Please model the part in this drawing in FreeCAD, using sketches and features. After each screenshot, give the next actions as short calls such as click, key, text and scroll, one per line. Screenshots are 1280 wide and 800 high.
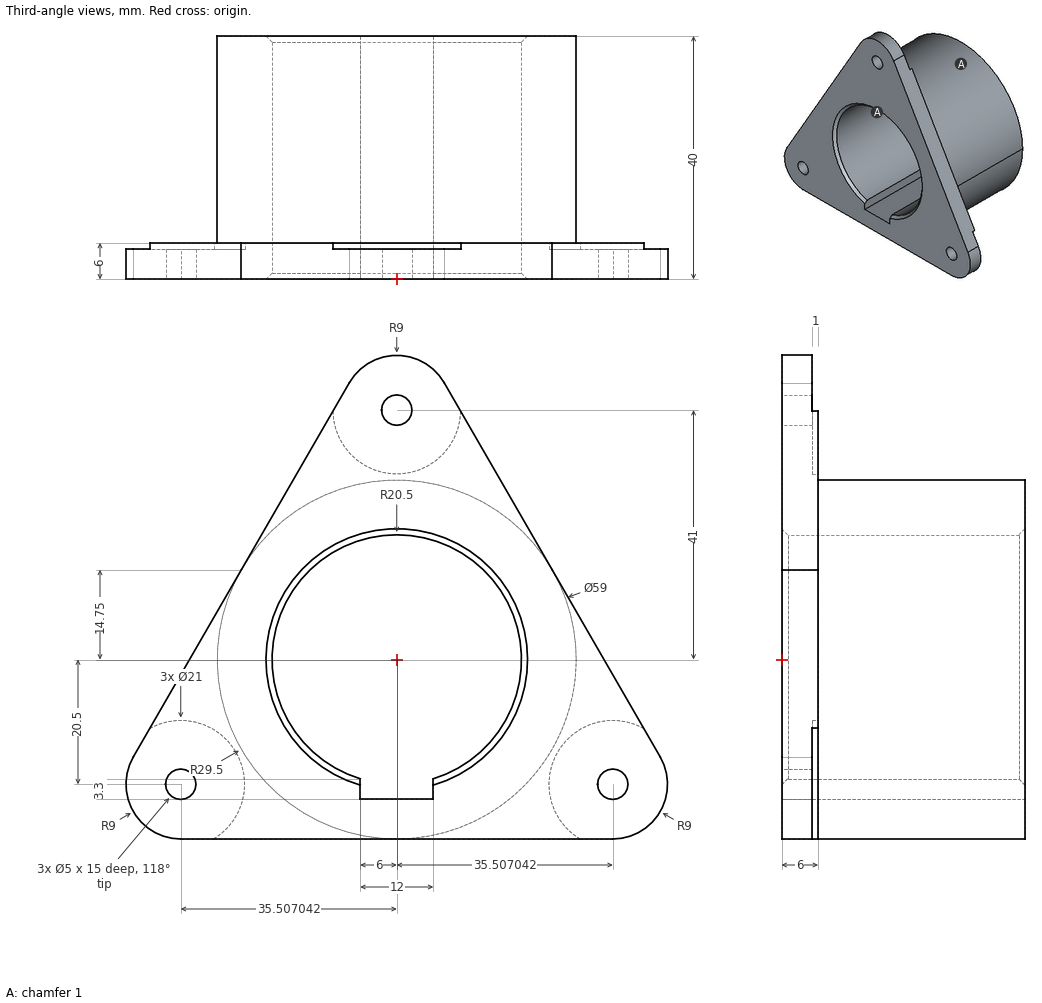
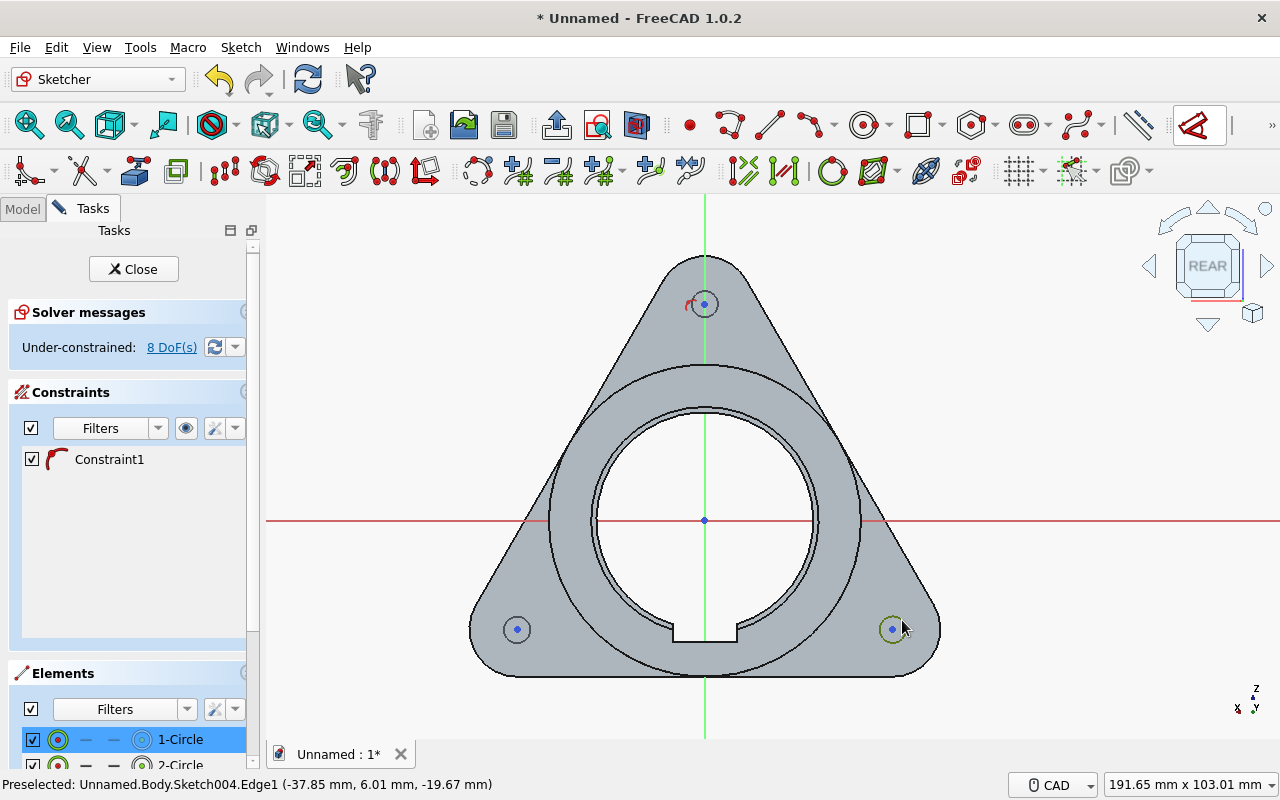
click(526, 621)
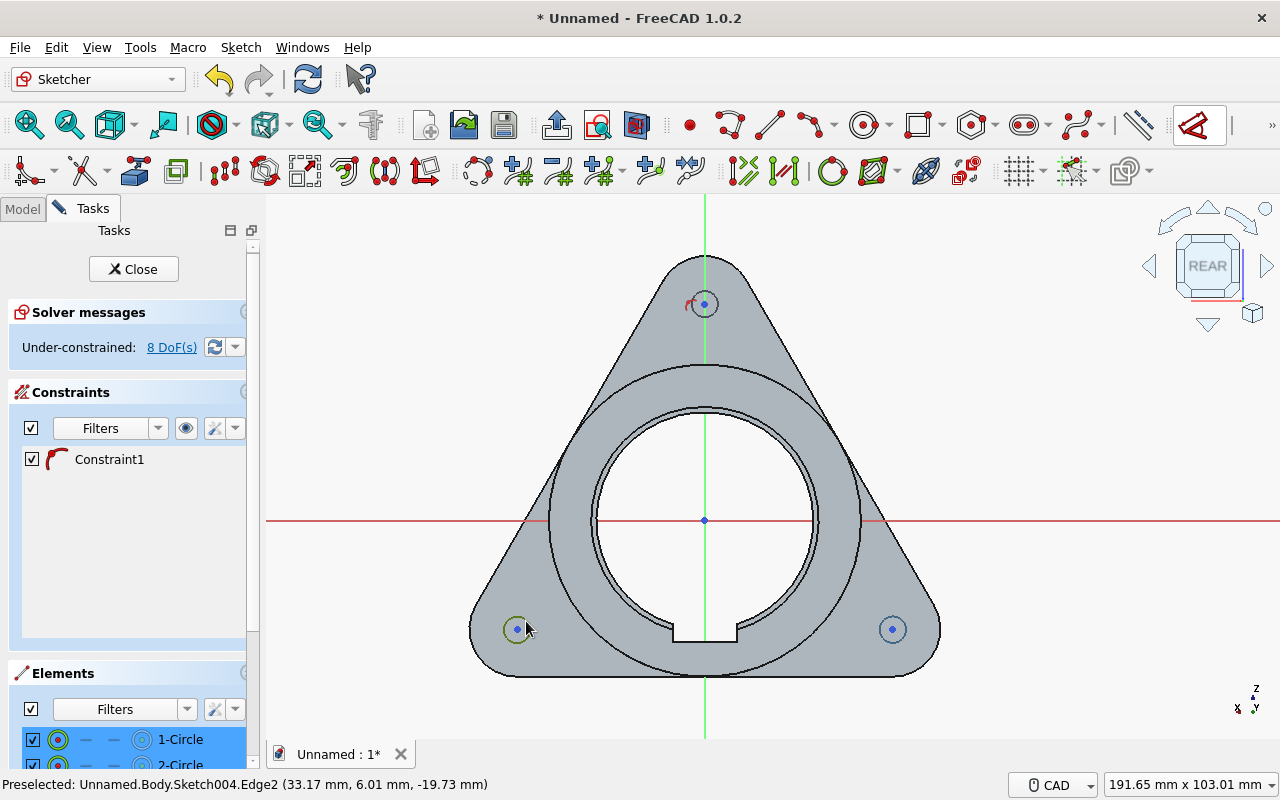
scroll(714, 295, up, 3)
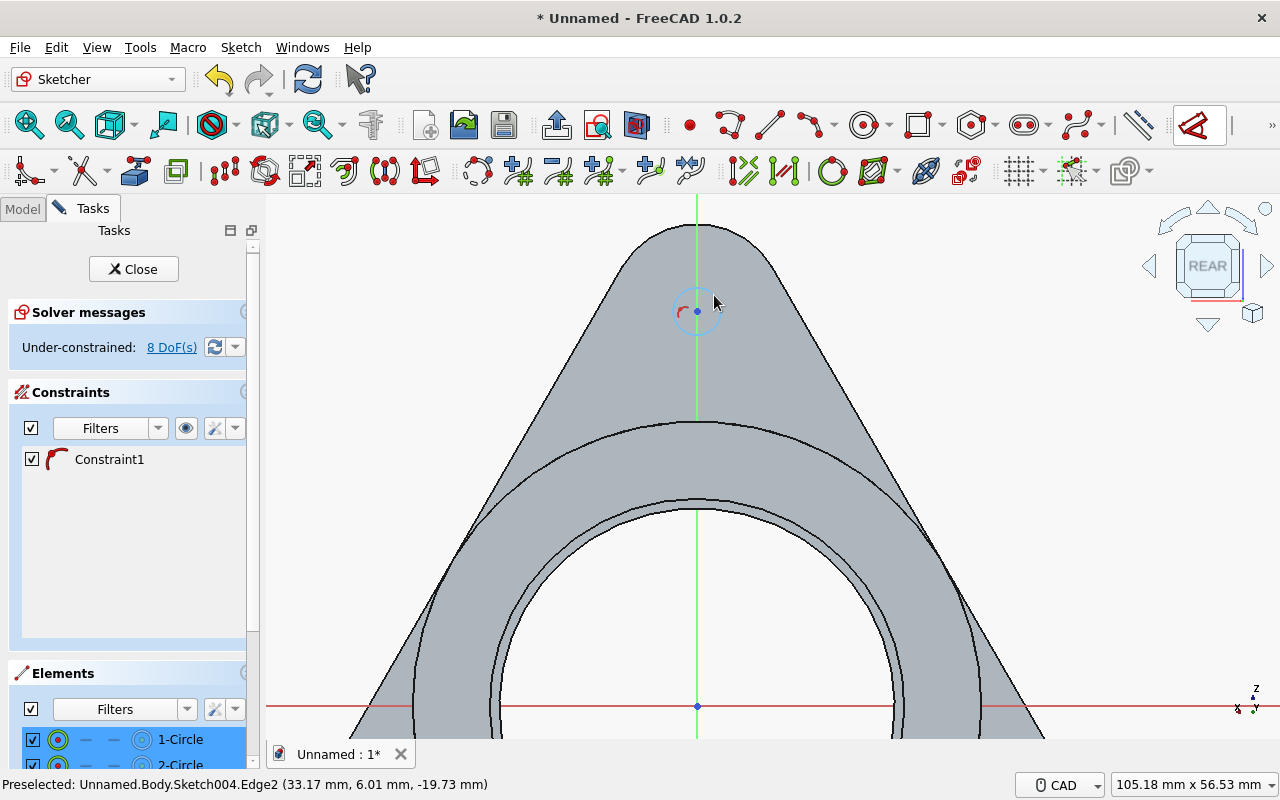
click(714, 295)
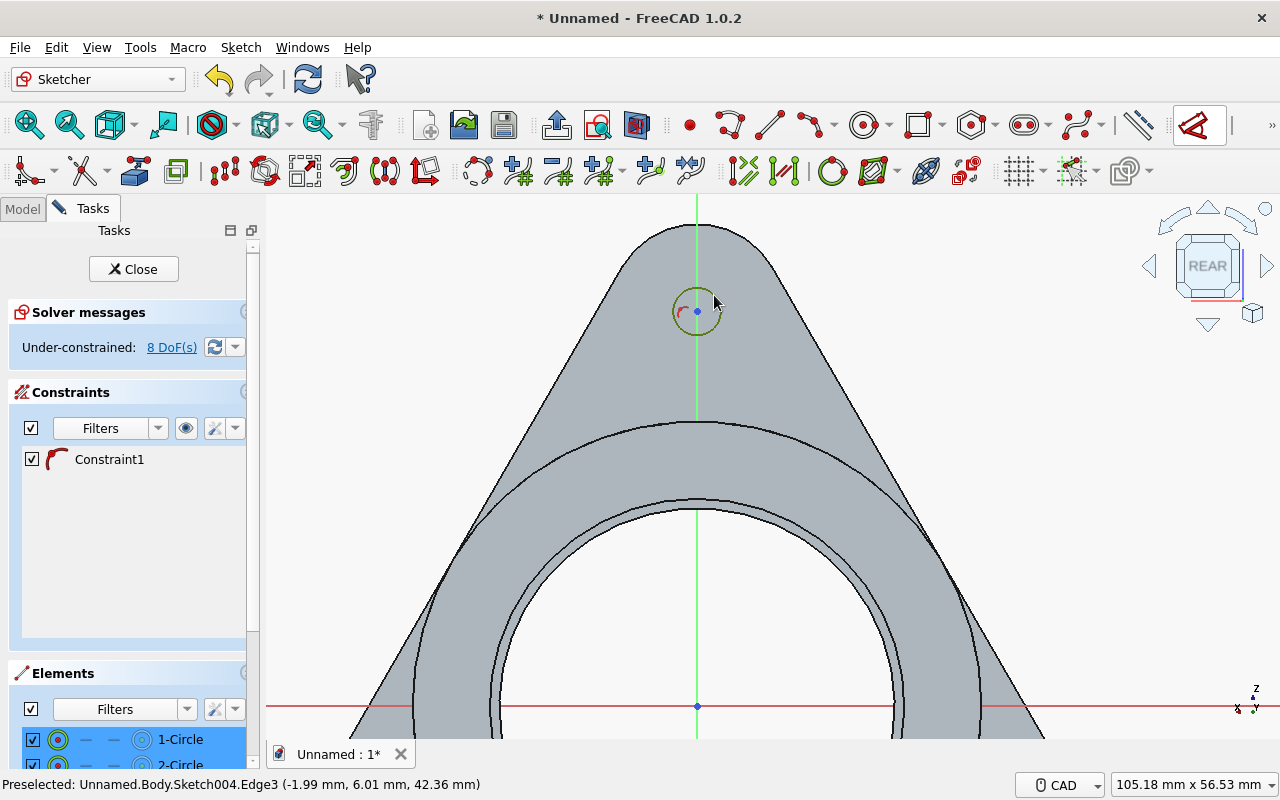
key(e)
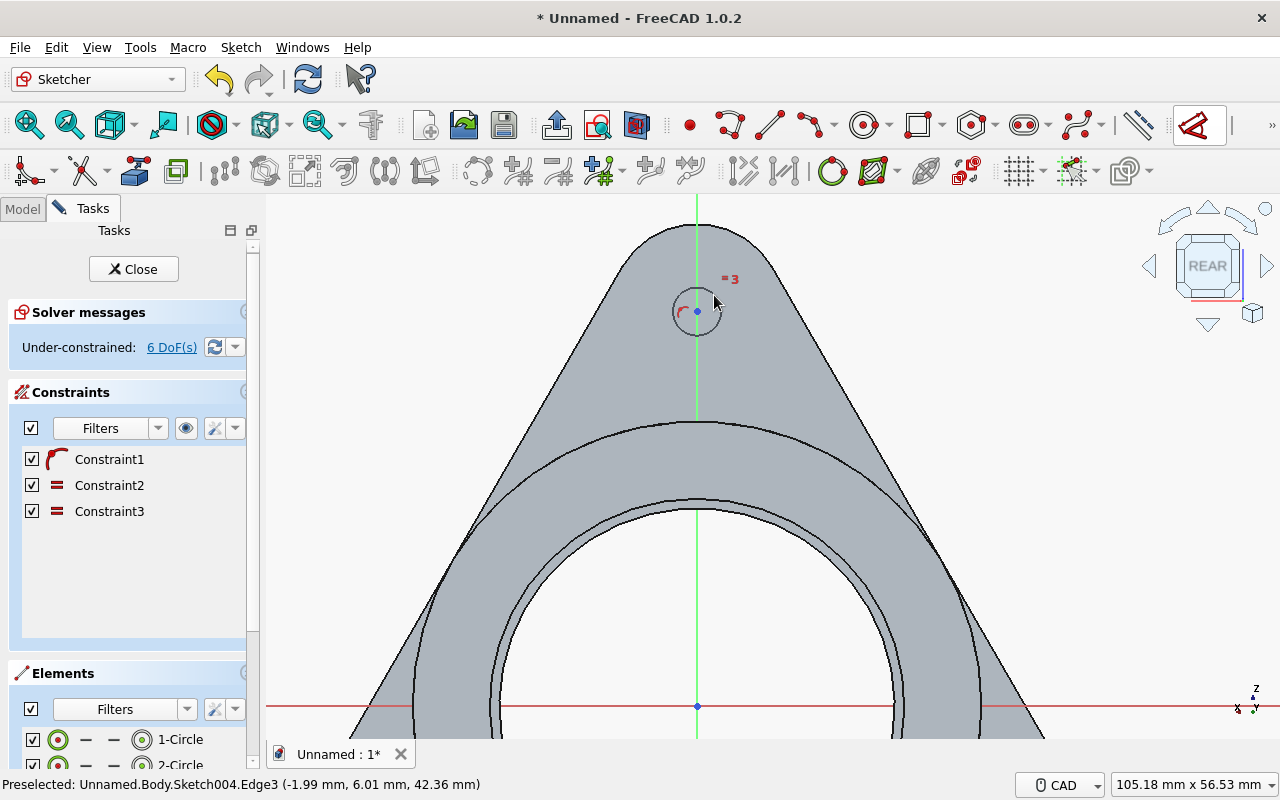
scroll(714, 295, down, 3)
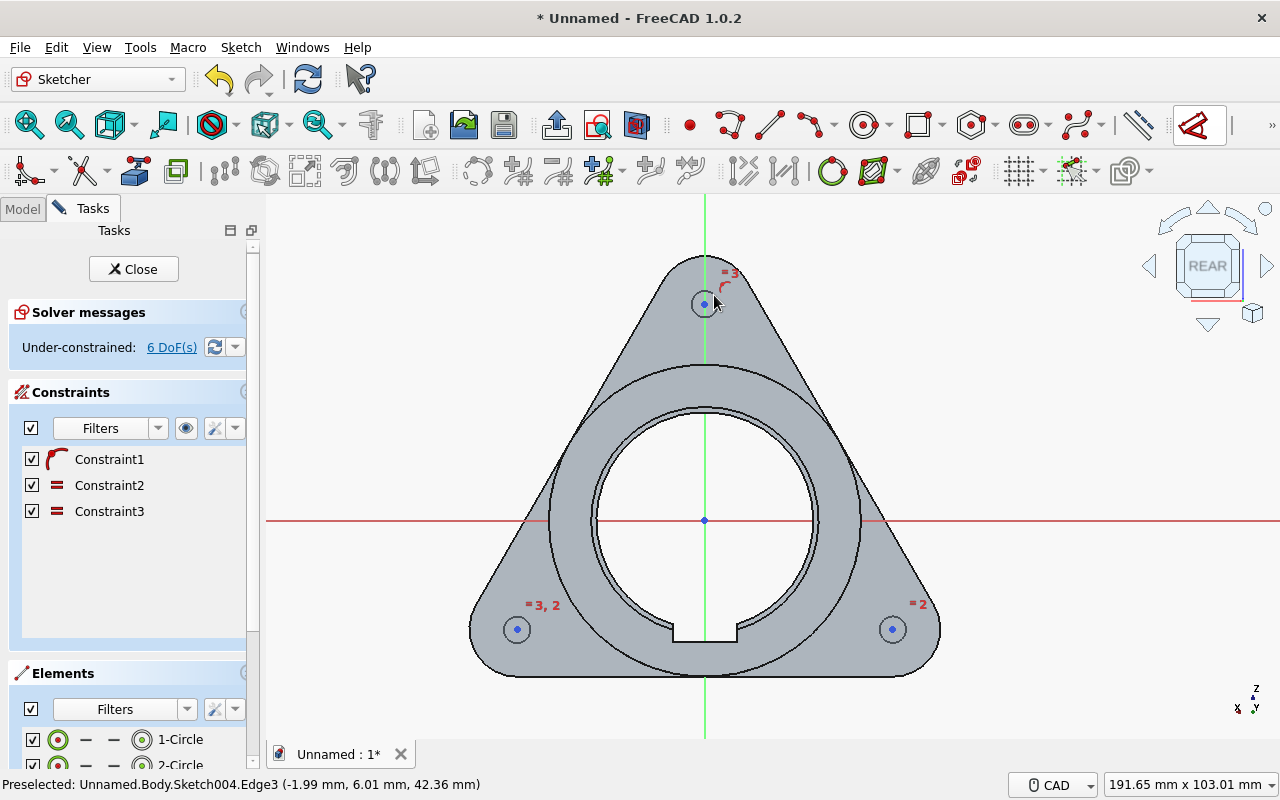
click(893, 630)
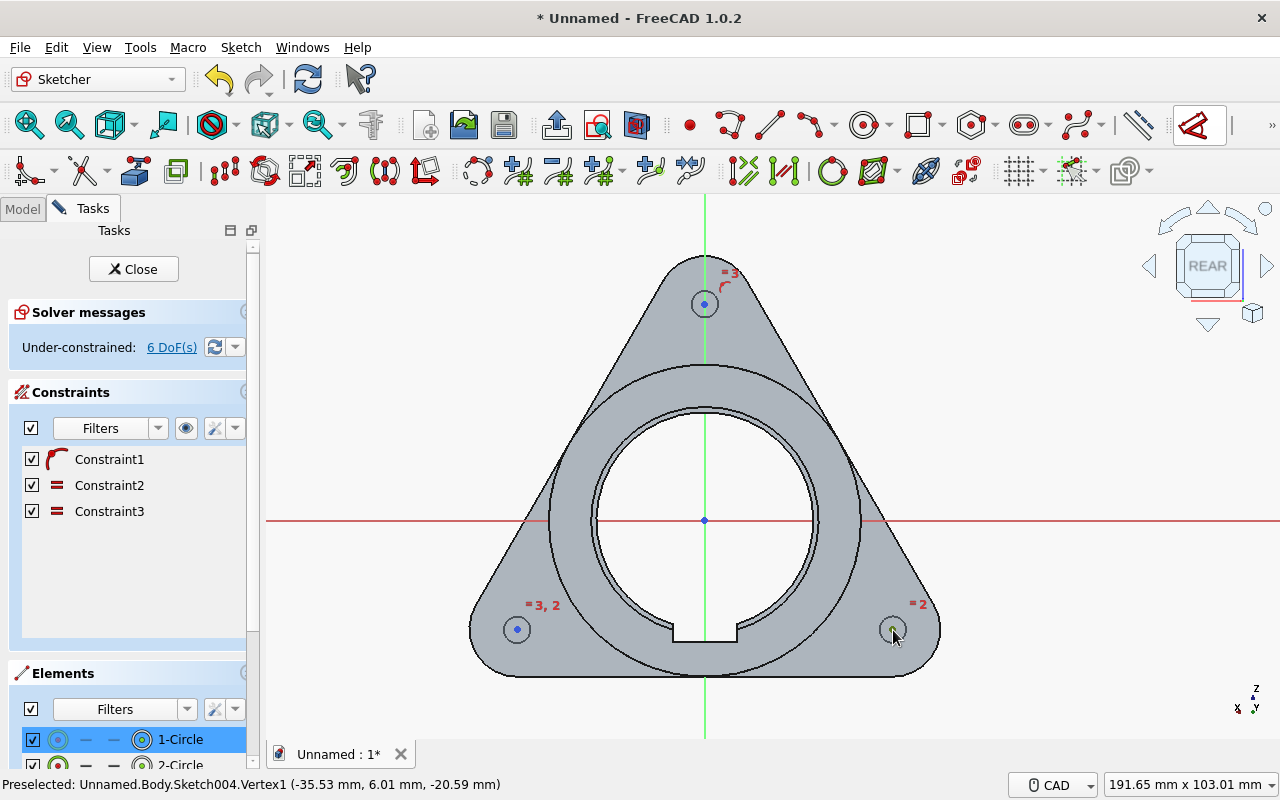
click(517, 630)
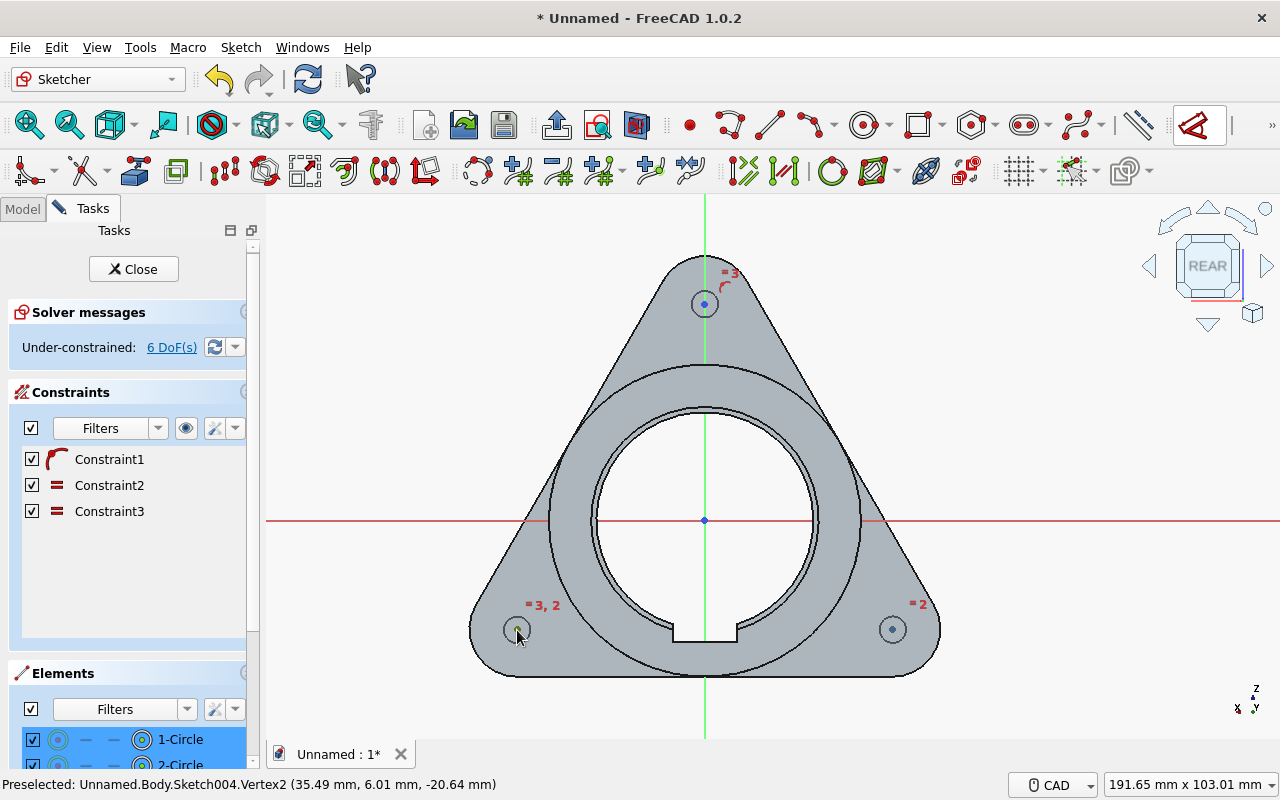
key(h)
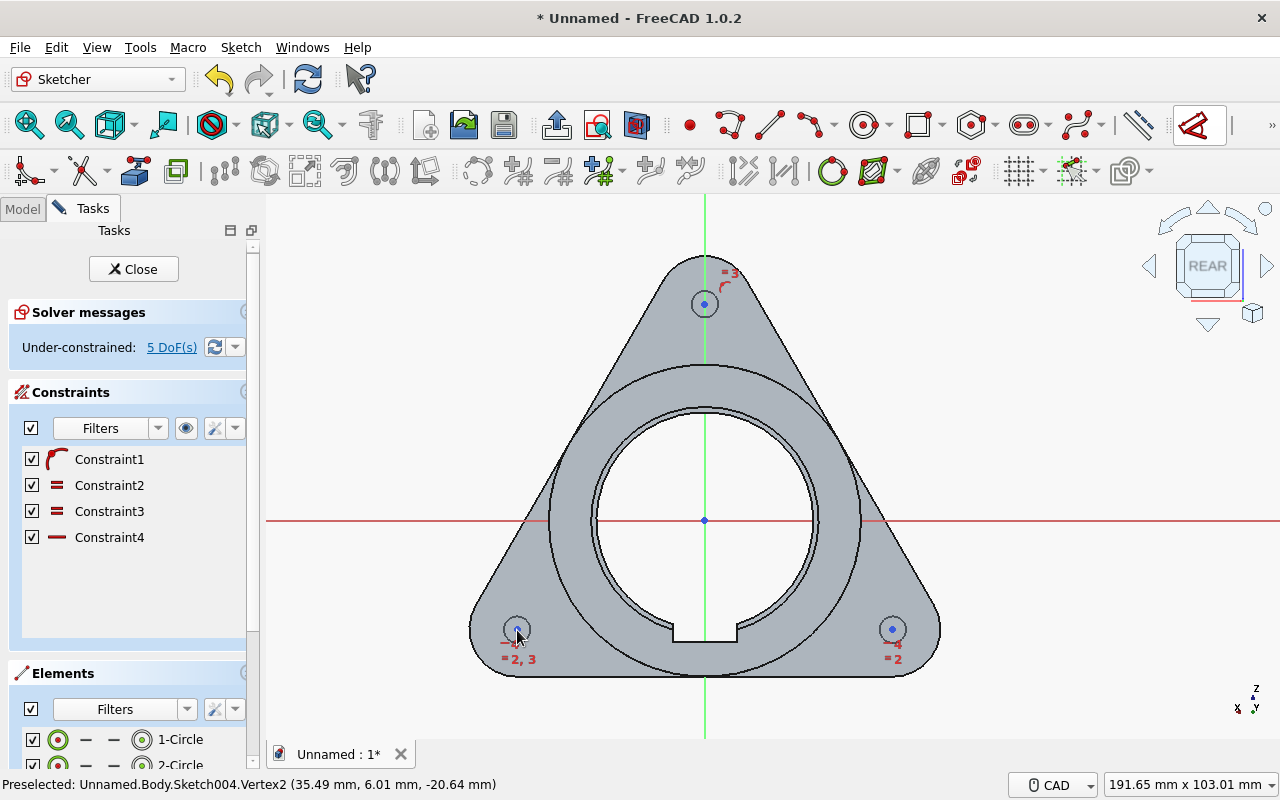
scroll(902, 620, up, 3)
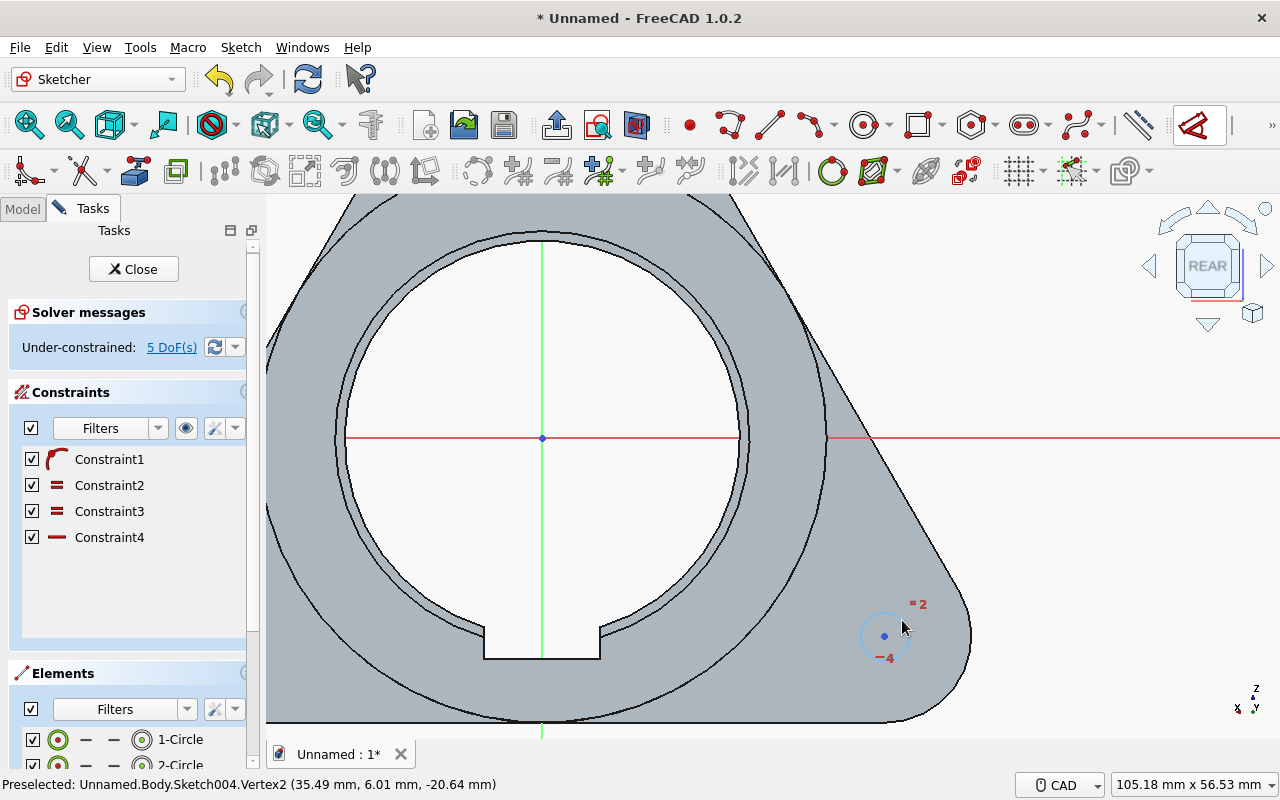
click(902, 620)